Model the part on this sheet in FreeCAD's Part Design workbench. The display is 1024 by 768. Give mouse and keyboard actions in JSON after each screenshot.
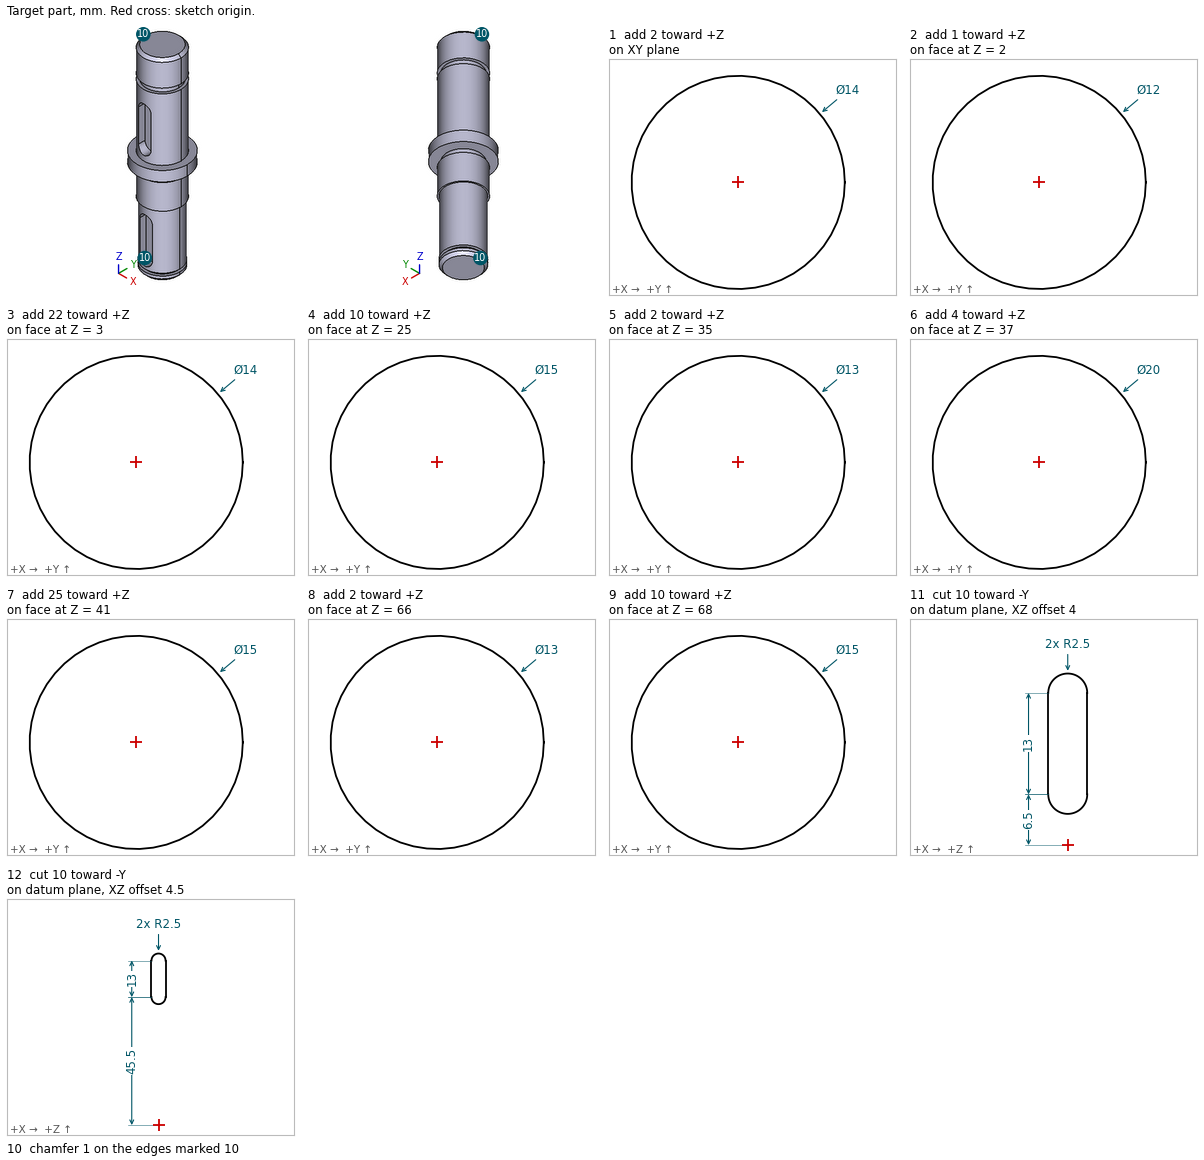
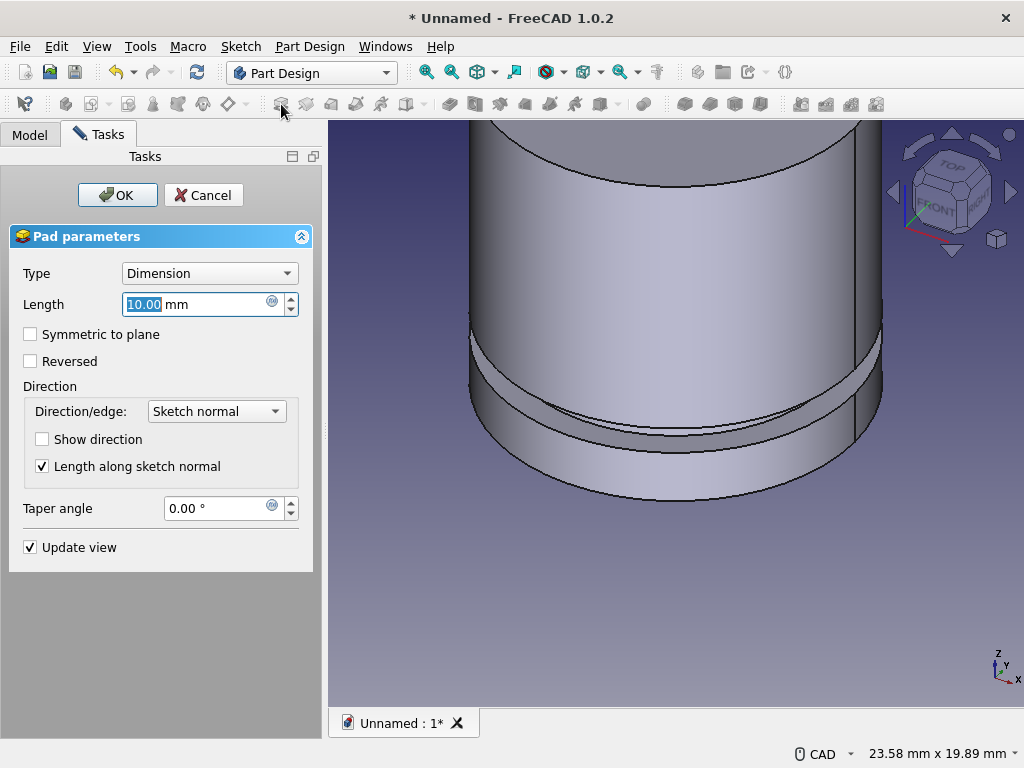
{"action": "type", "text": "22"}
{"action": "key", "text": "Tab"}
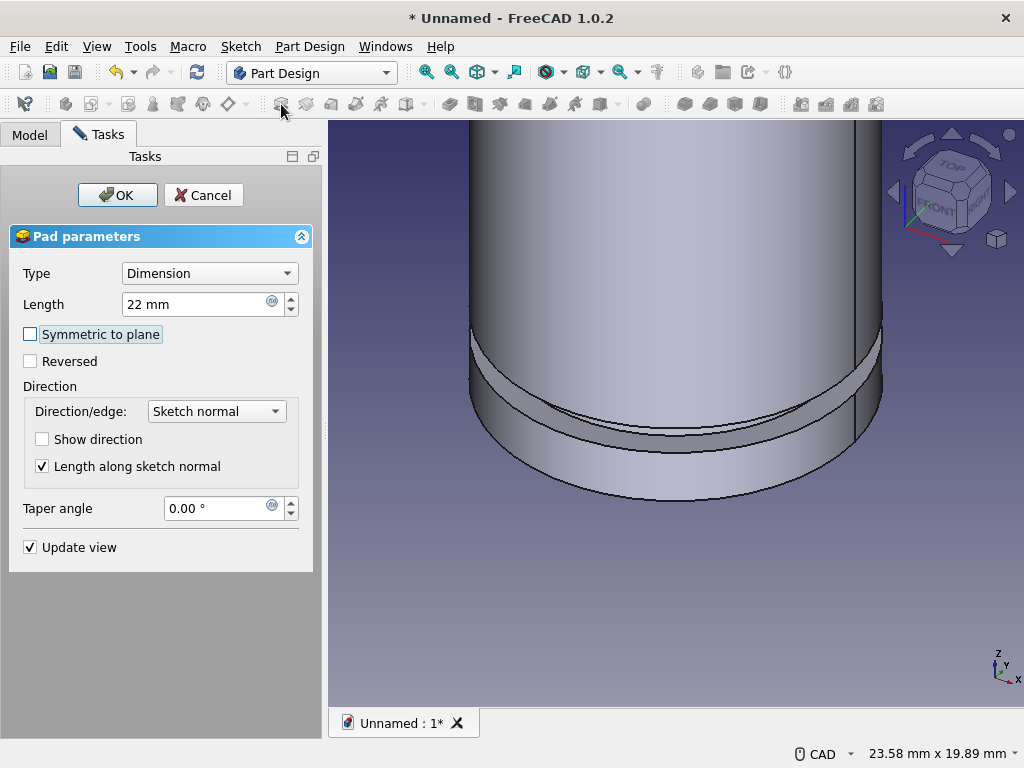
{"action": "left_click", "coordinate": [118, 195]}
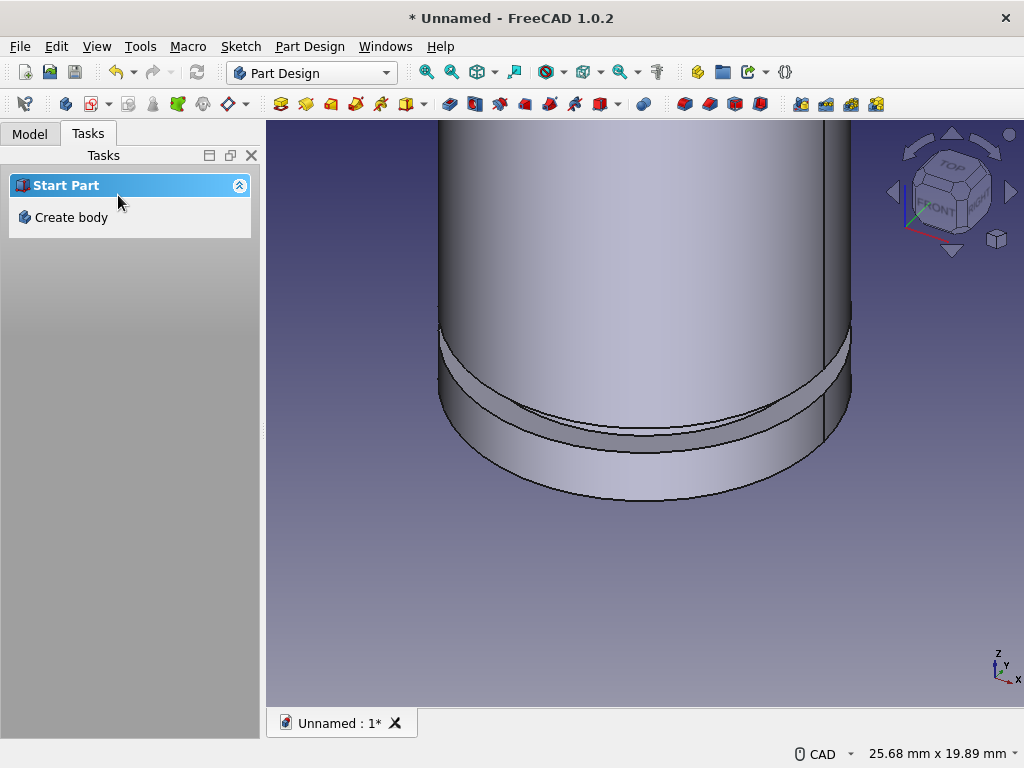
{"action": "key", "text": "v f"}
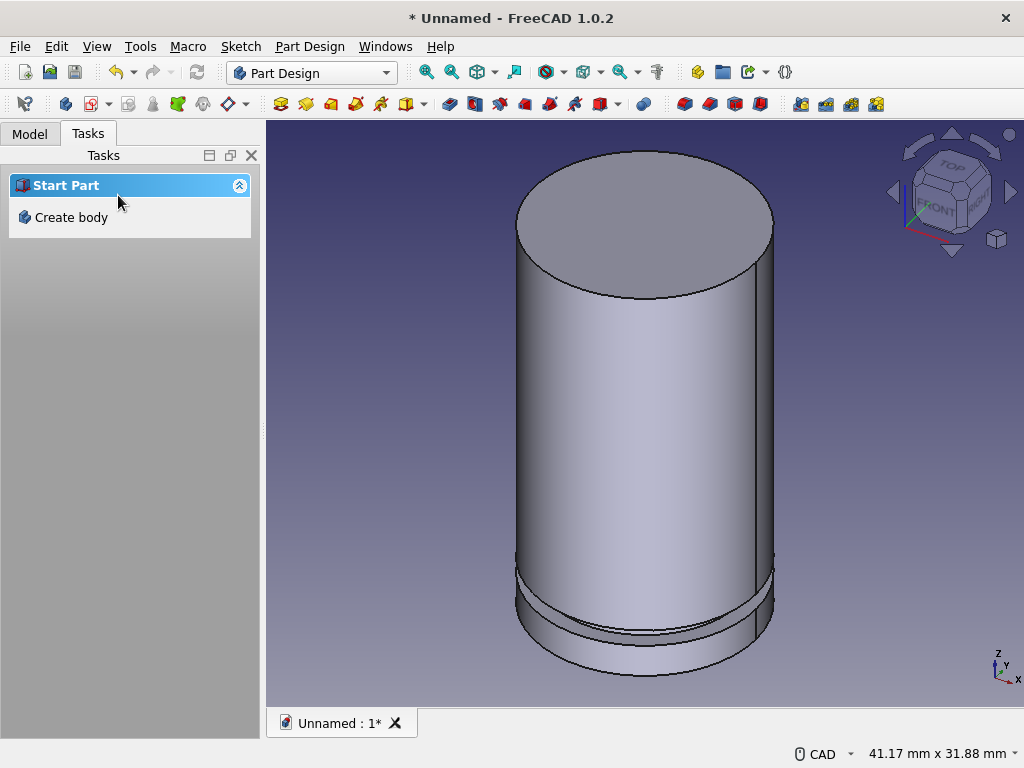
{"action": "left_click", "coordinate": [645, 224]}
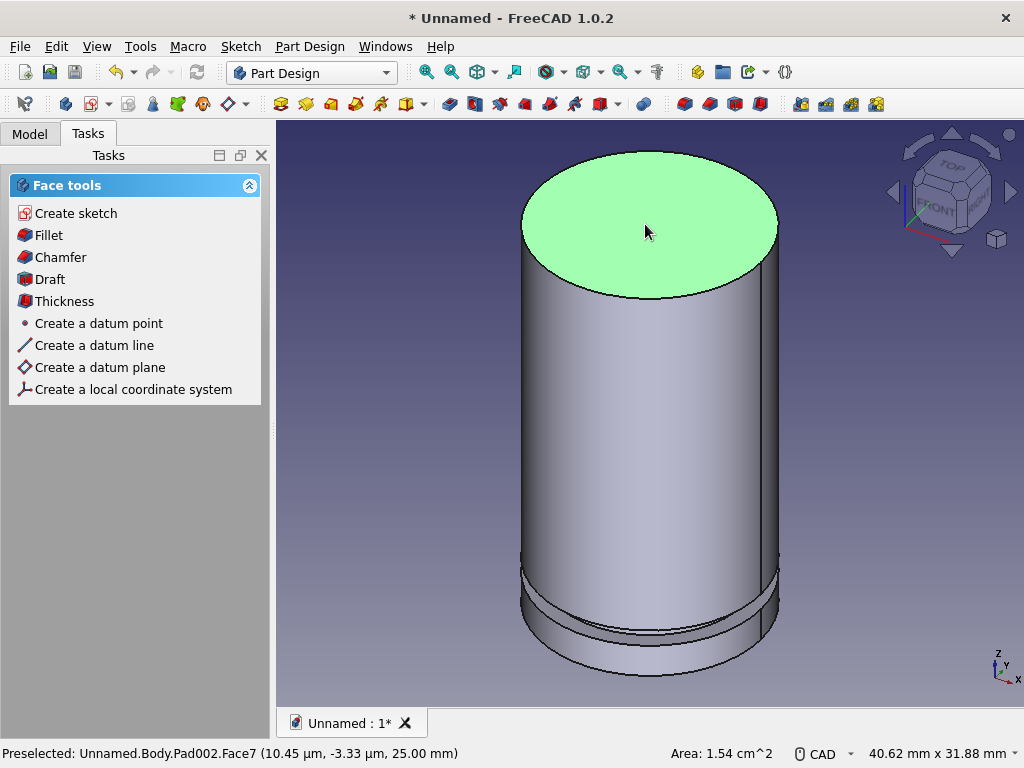
{"action": "left_click", "coordinate": [90, 104]}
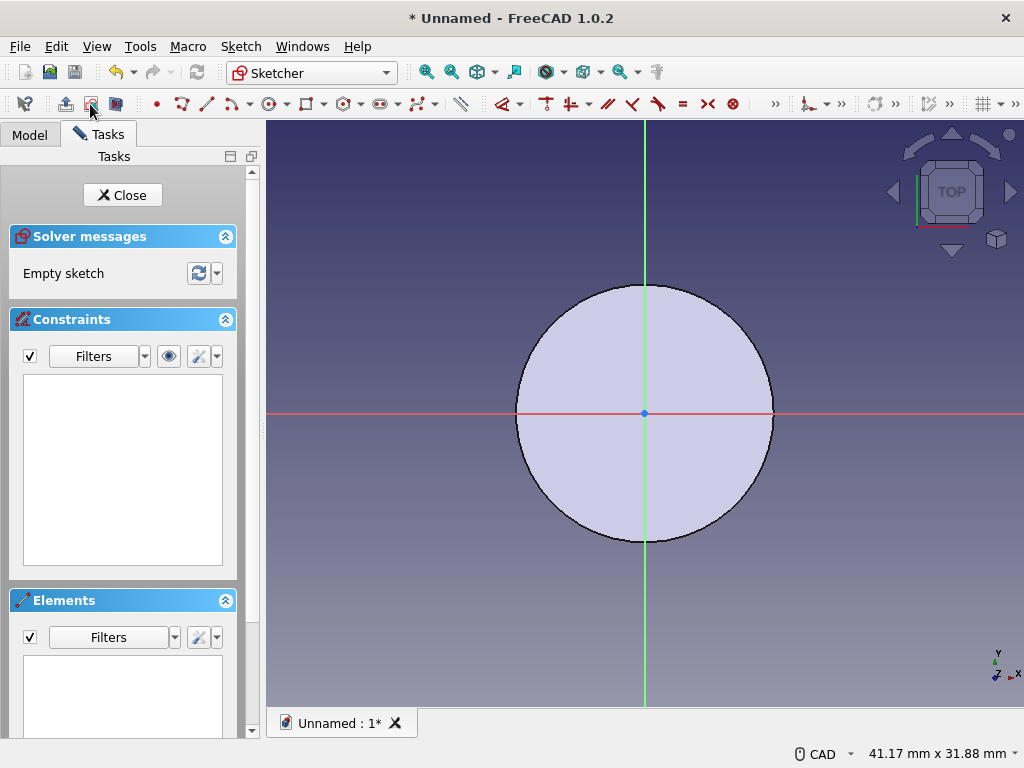
{"action": "scroll", "coordinate": [784, 413], "scroll_direction": "up", "scroll_amount": 2}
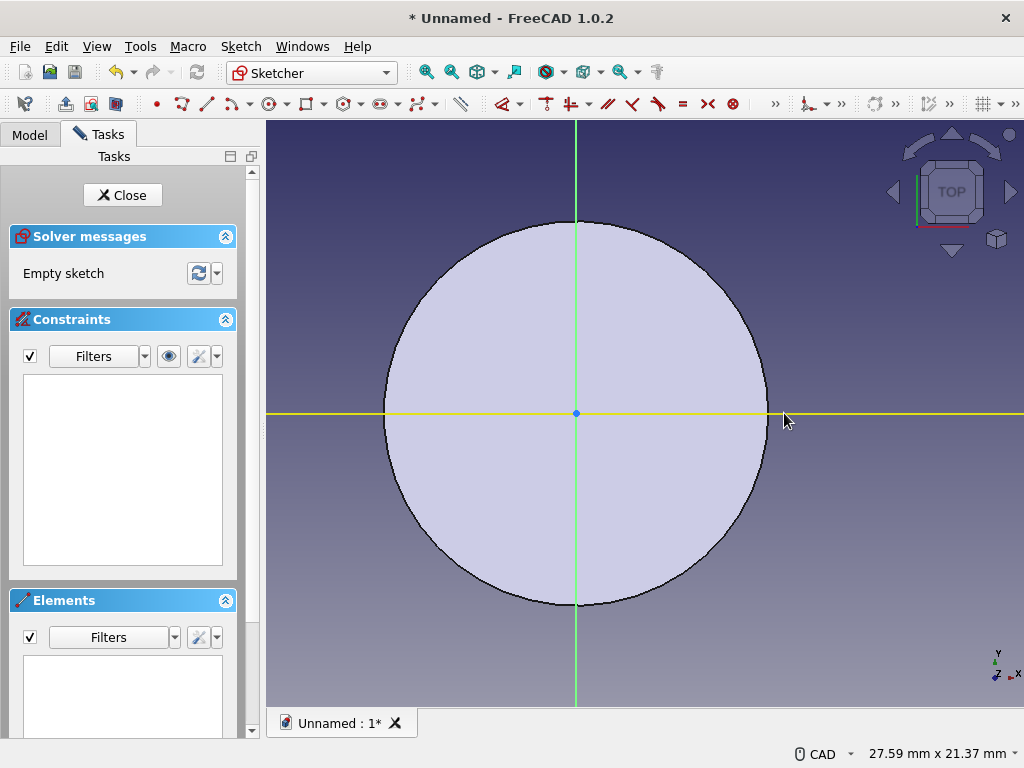
{"action": "left_click", "coordinate": [268, 104]}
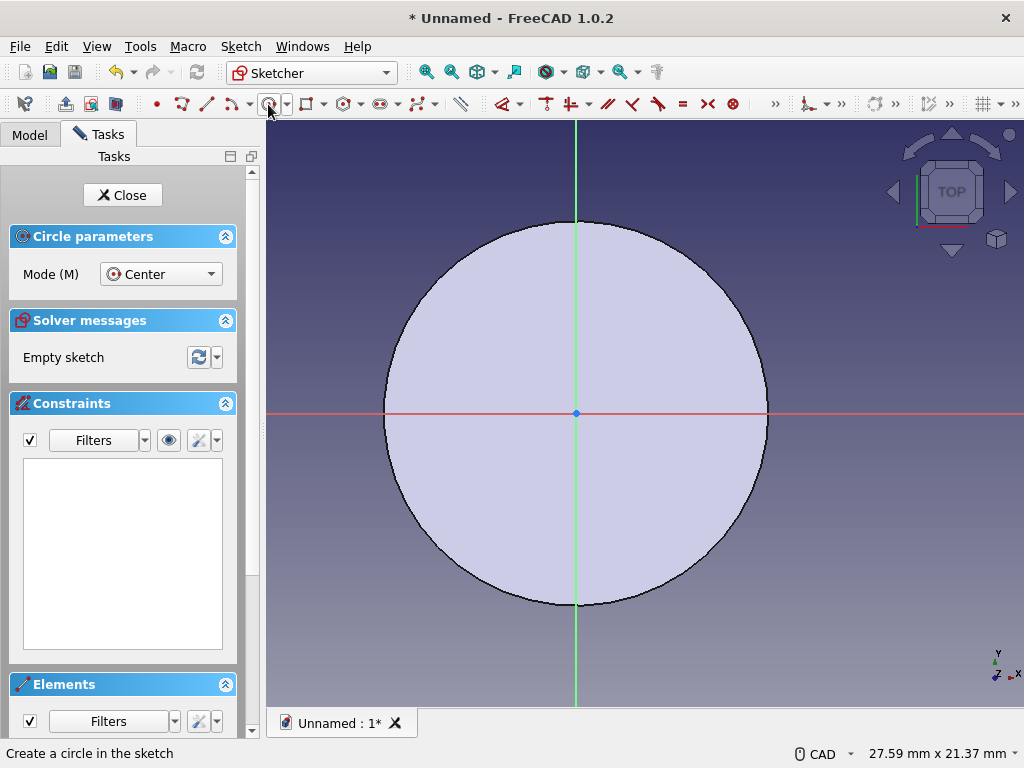
{"action": "left_click", "coordinate": [576, 414]}
{"action": "left_click", "coordinate": [722, 268]}
{"action": "key", "text": "Escape"}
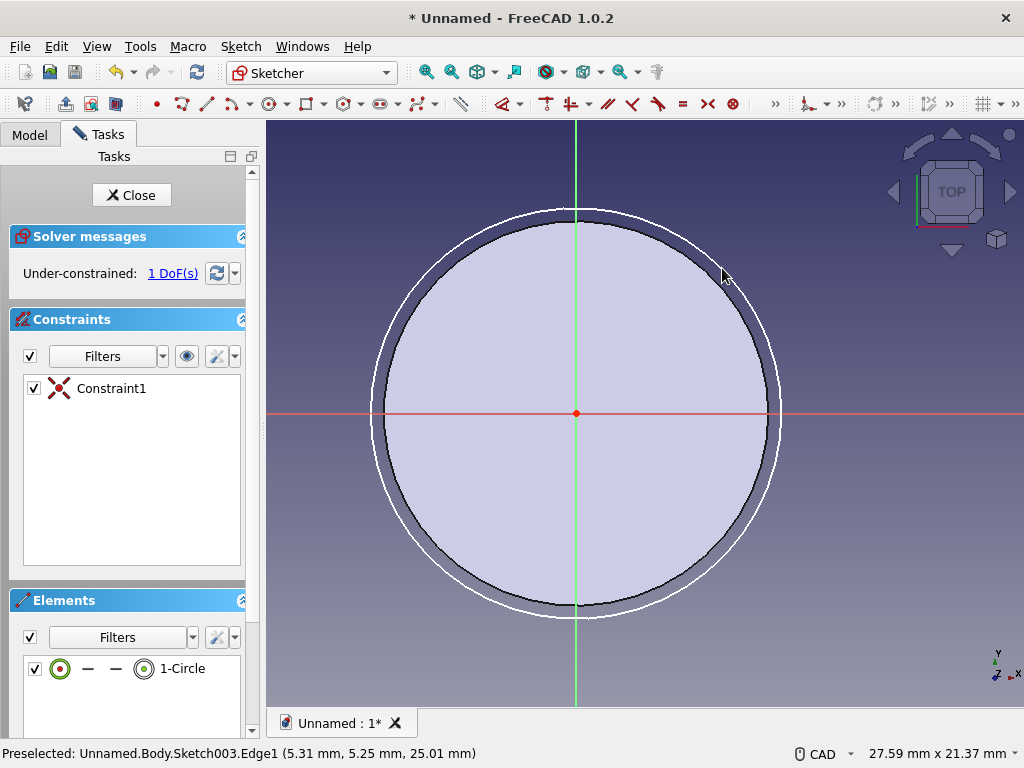
{"action": "left_click", "coordinate": [502, 104]}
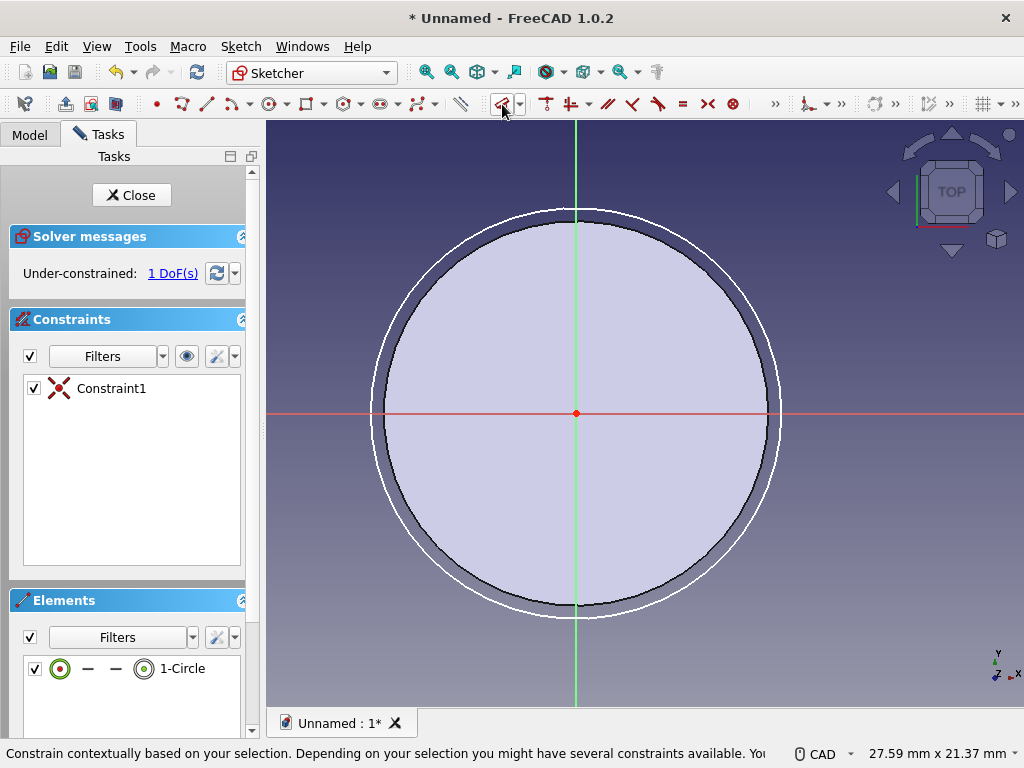
{"action": "left_click", "coordinate": [721, 268]}
{"action": "left_click", "coordinate": [744, 245]}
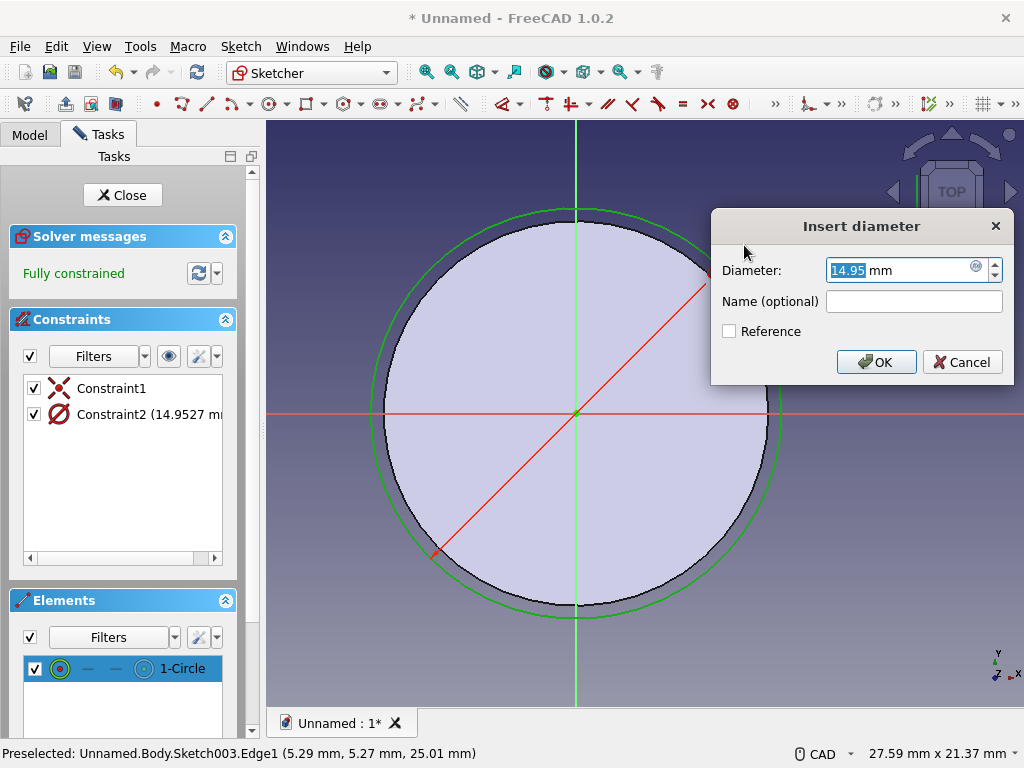
{"action": "type", "text": "15"}
{"action": "key", "text": "Return"}
{"action": "key", "text": "Escape"}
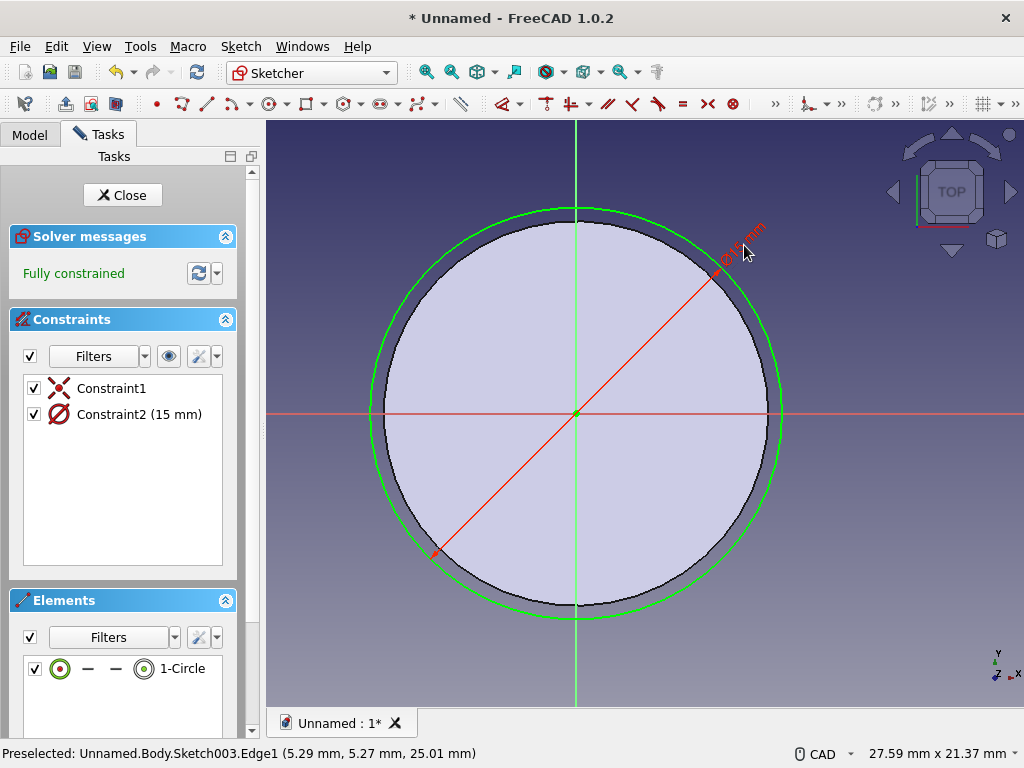
{"action": "left_click", "coordinate": [123, 195]}